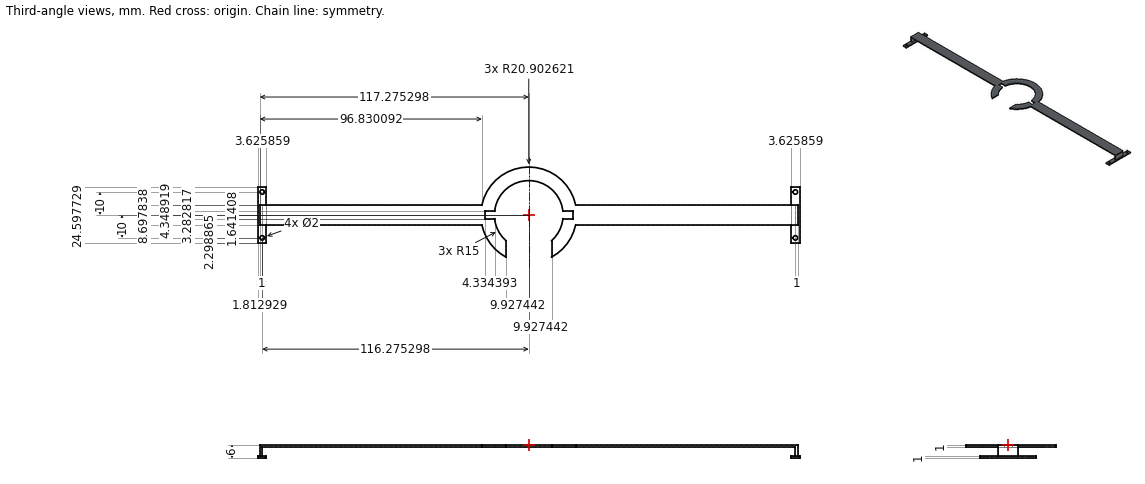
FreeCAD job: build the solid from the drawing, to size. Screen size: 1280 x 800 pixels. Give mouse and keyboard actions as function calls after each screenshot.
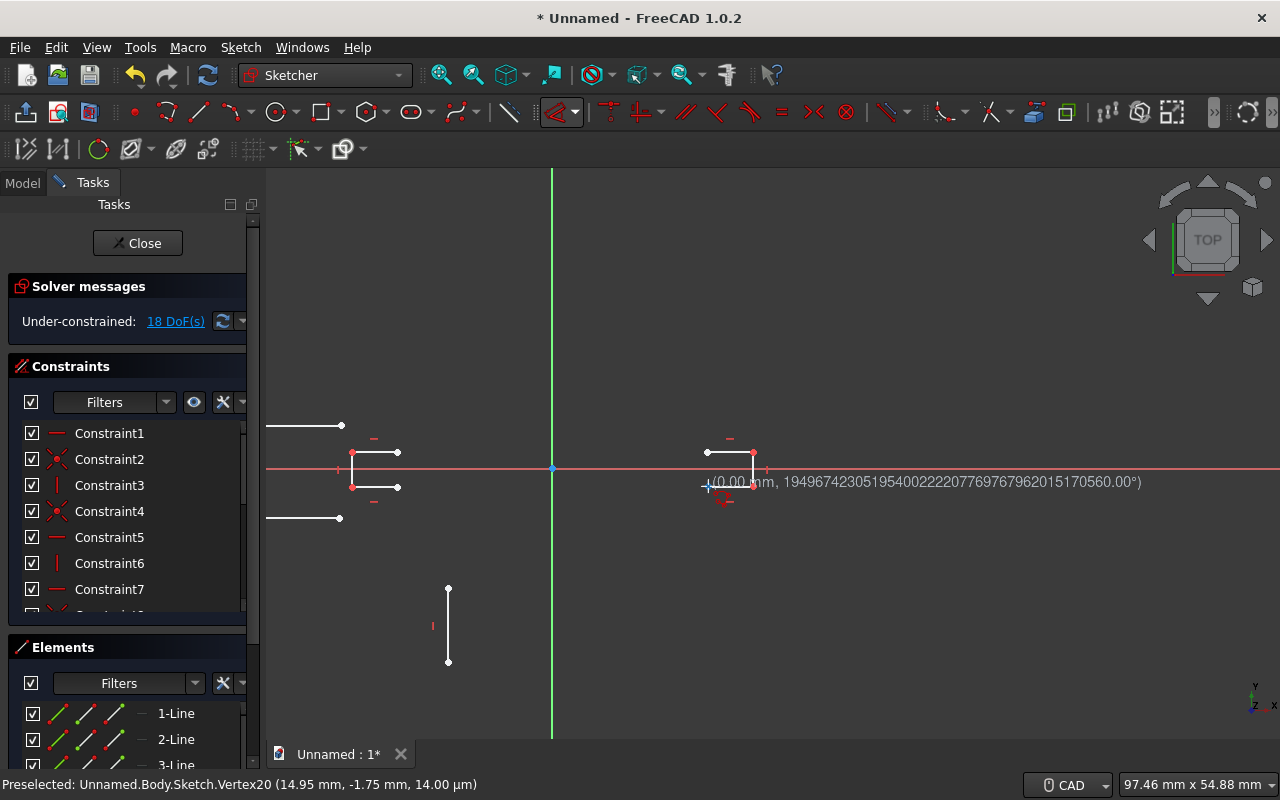
click(200, 112)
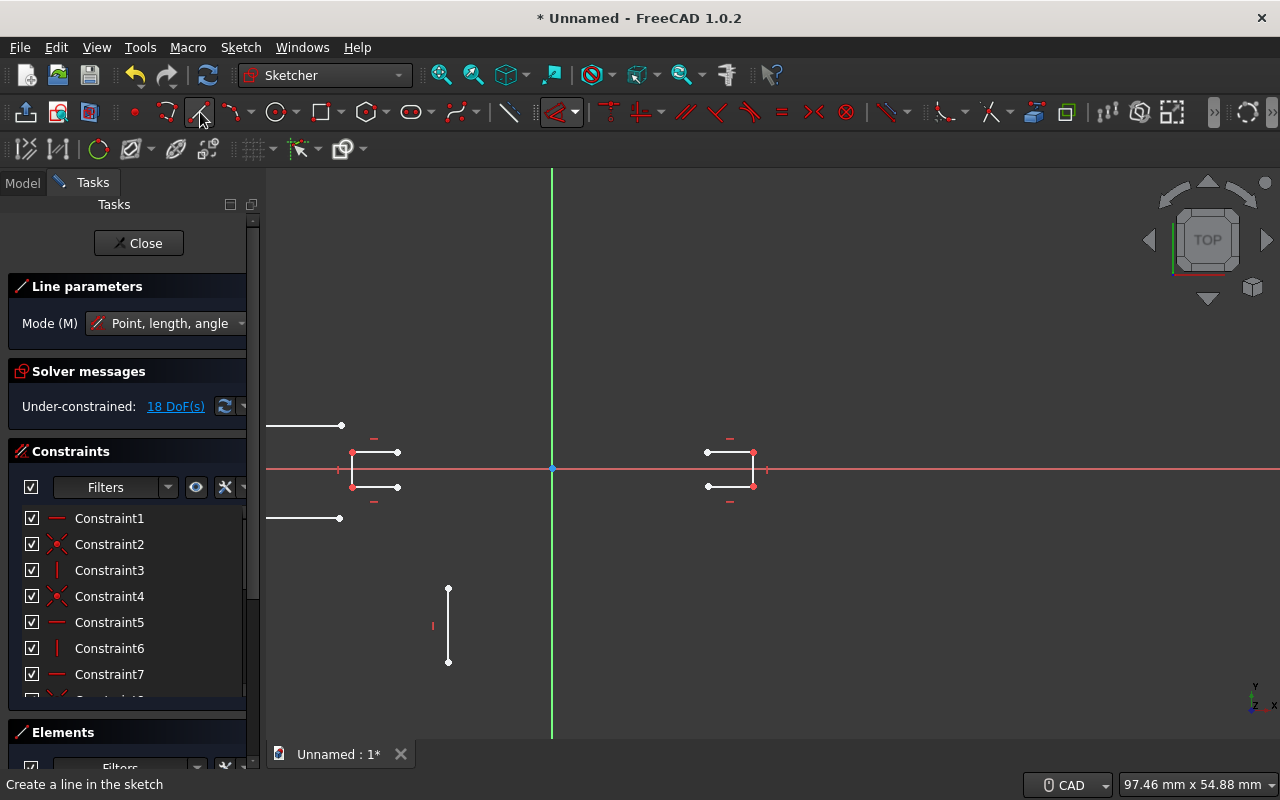
scroll(754, 453, down, 7)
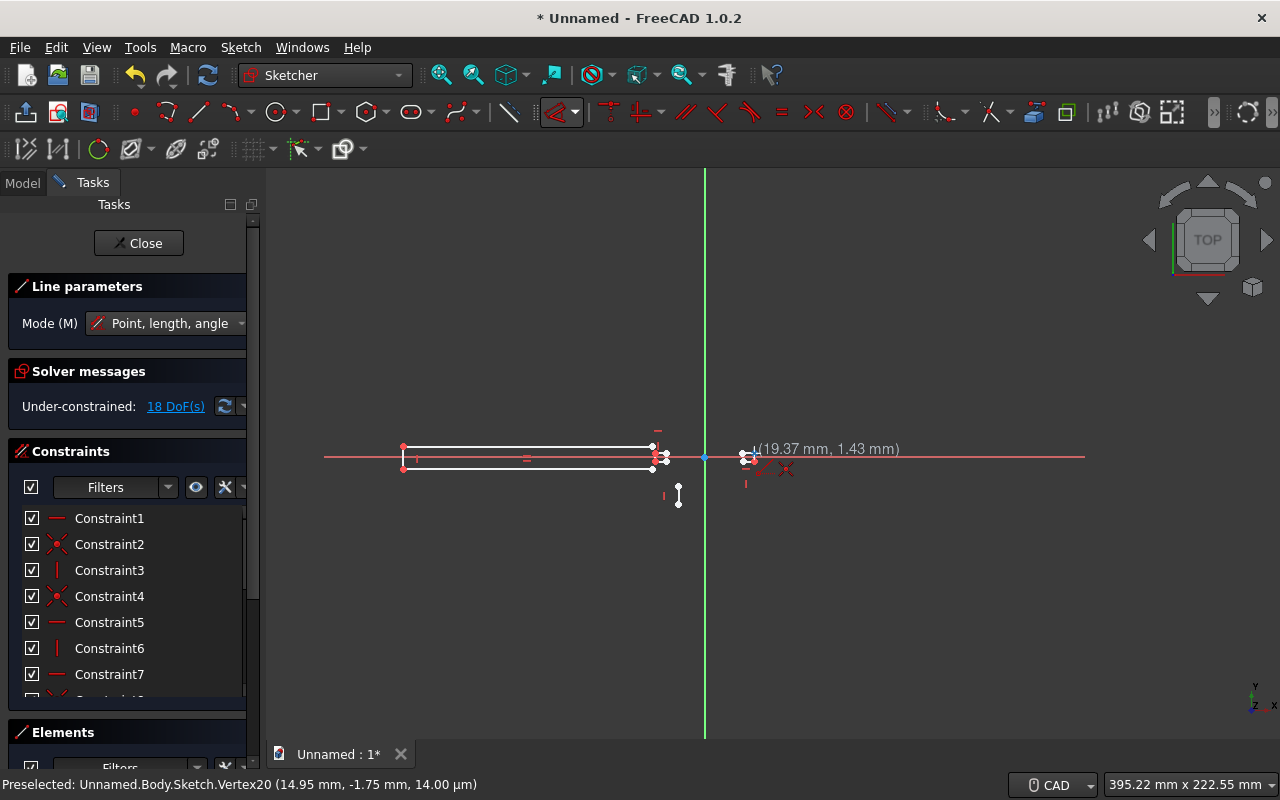
click(730, 486)
click(730, 504)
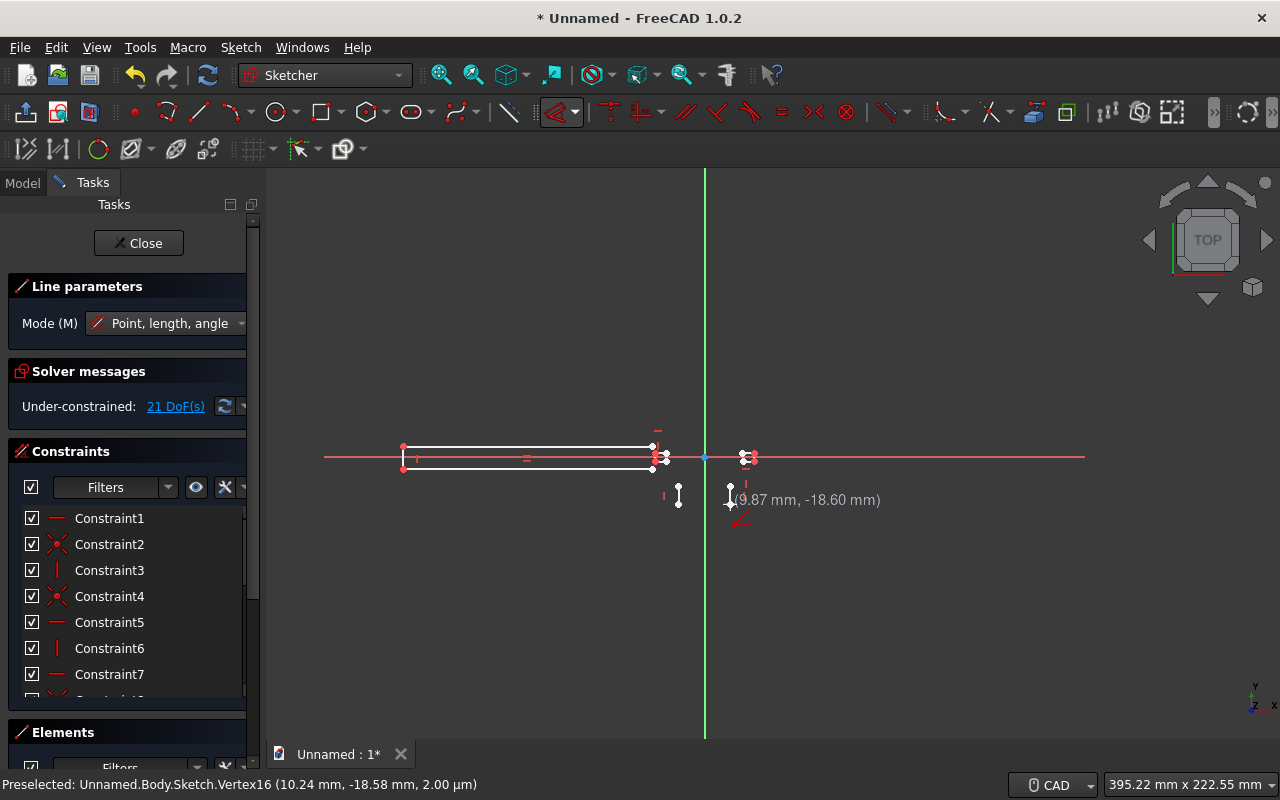
key(g)
key(m)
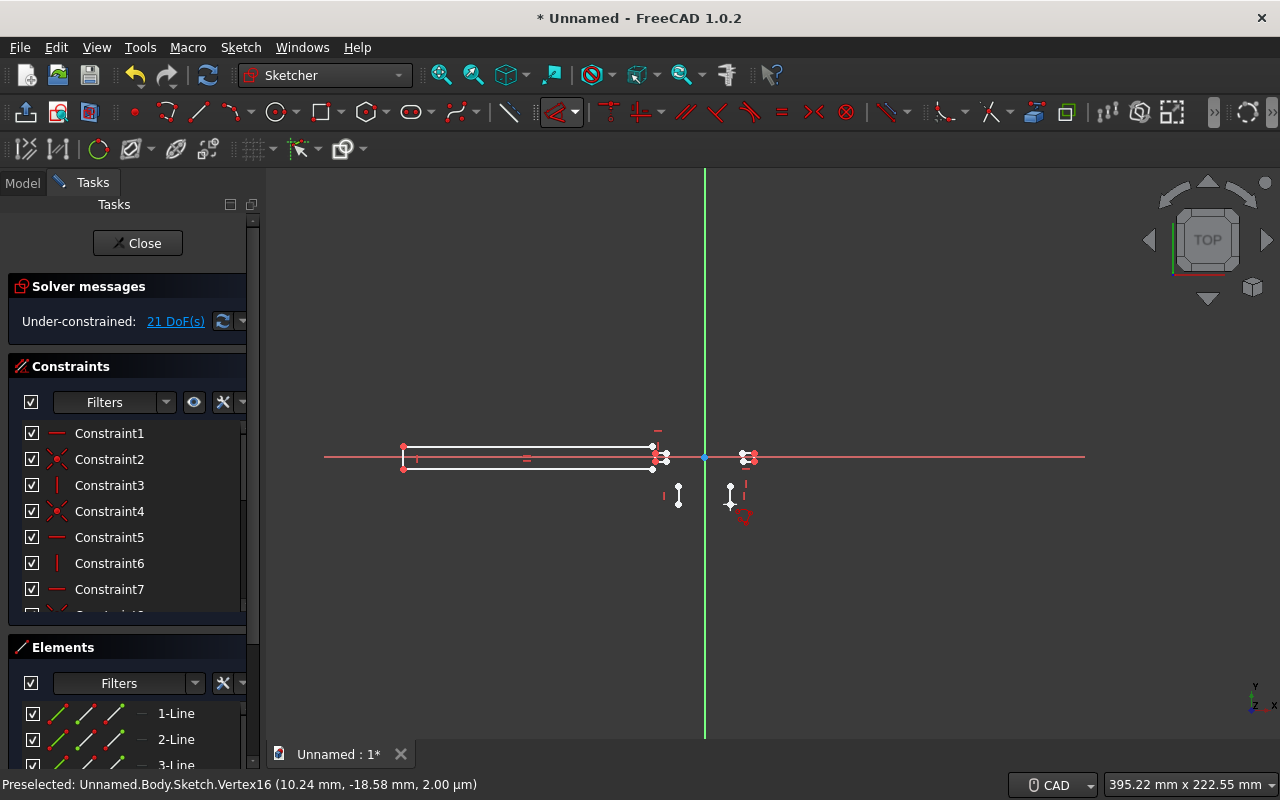
scroll(757, 468, up, 4)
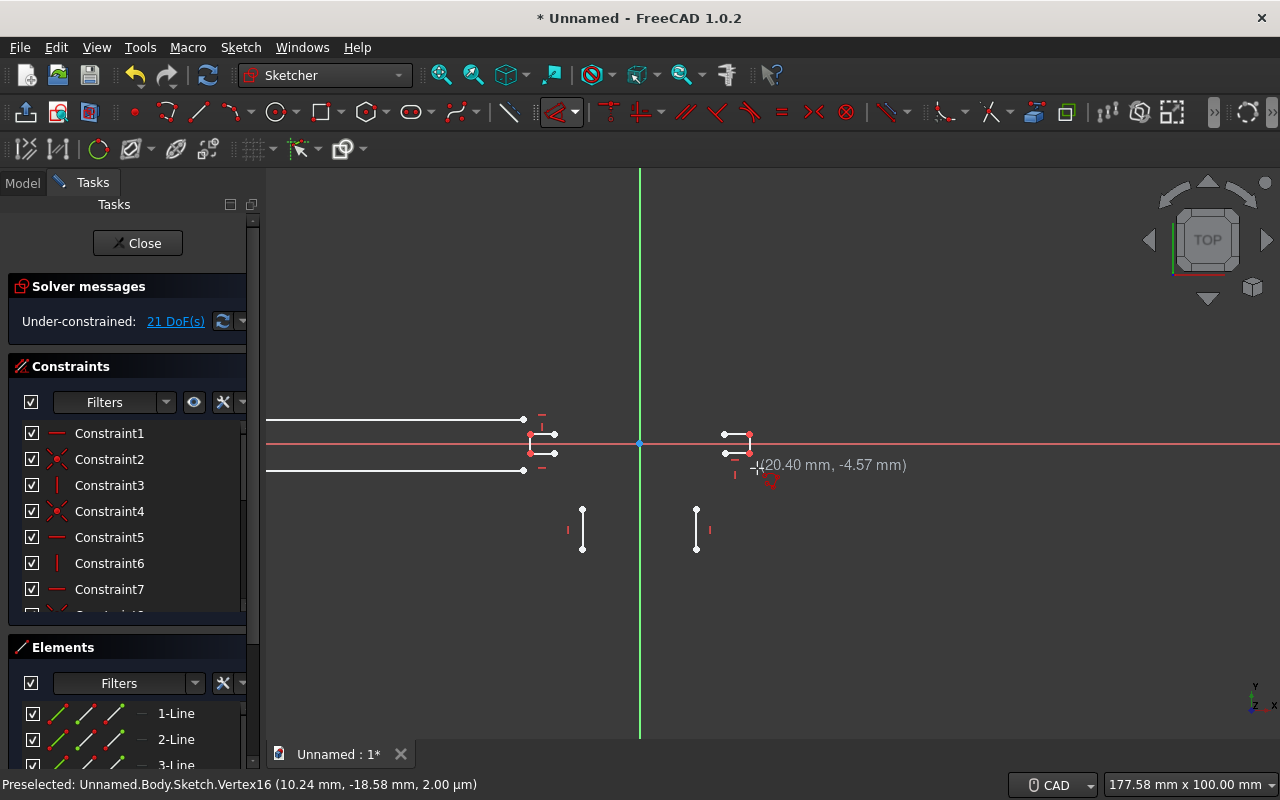
click(757, 468)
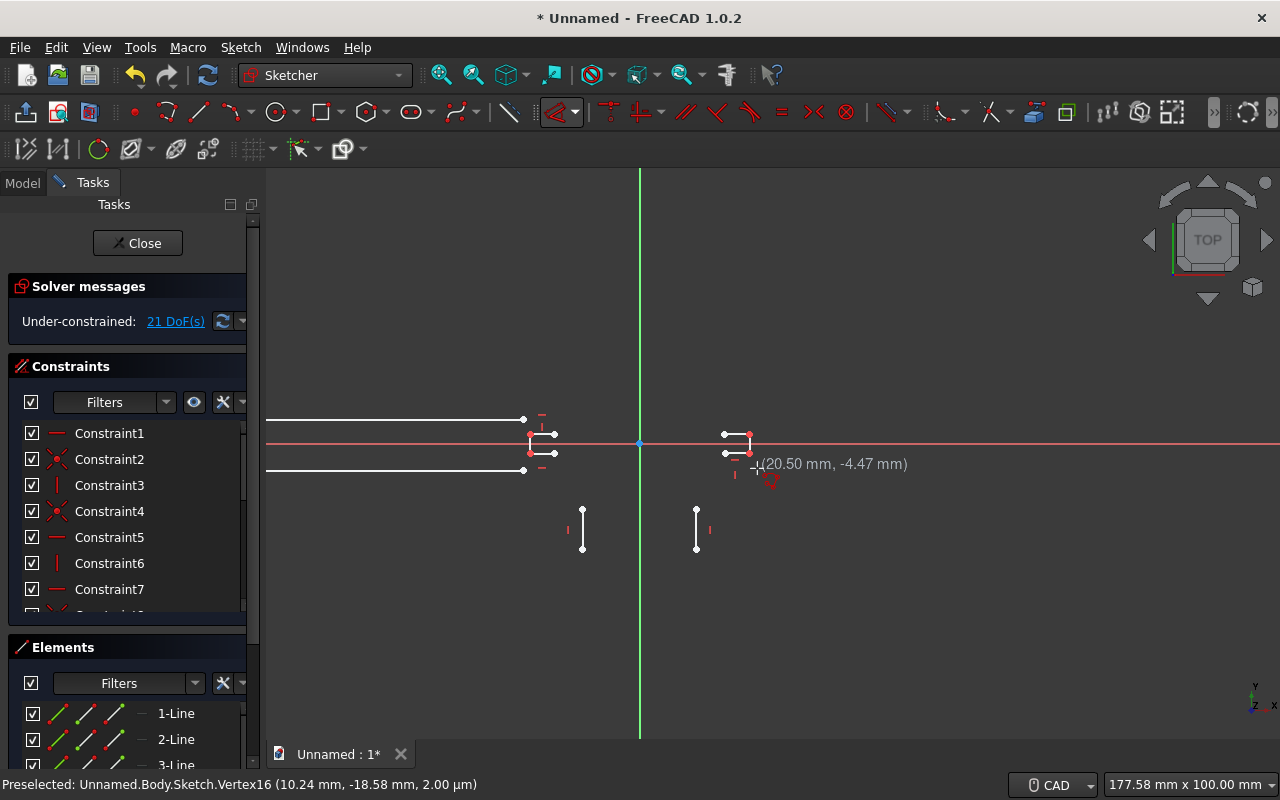
scroll(757, 467, down, 4)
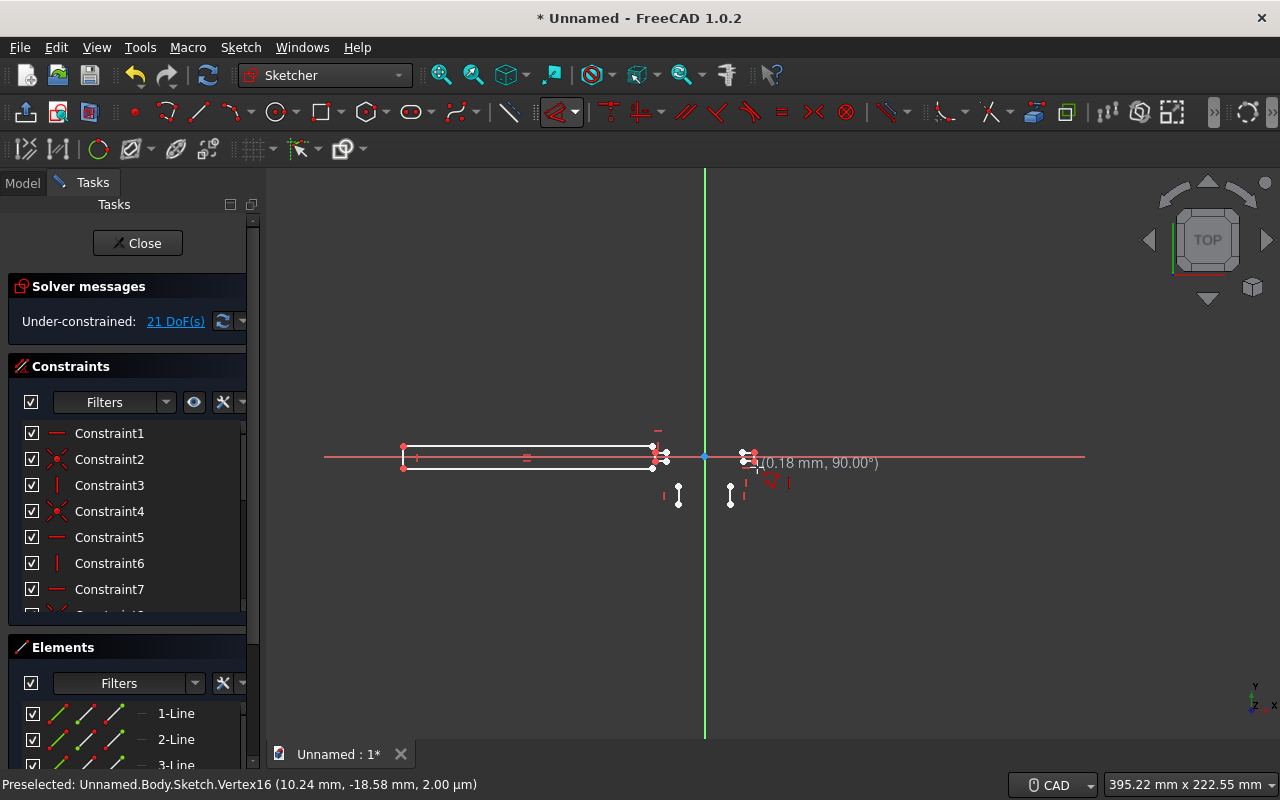
scroll(1006, 468, up, 2)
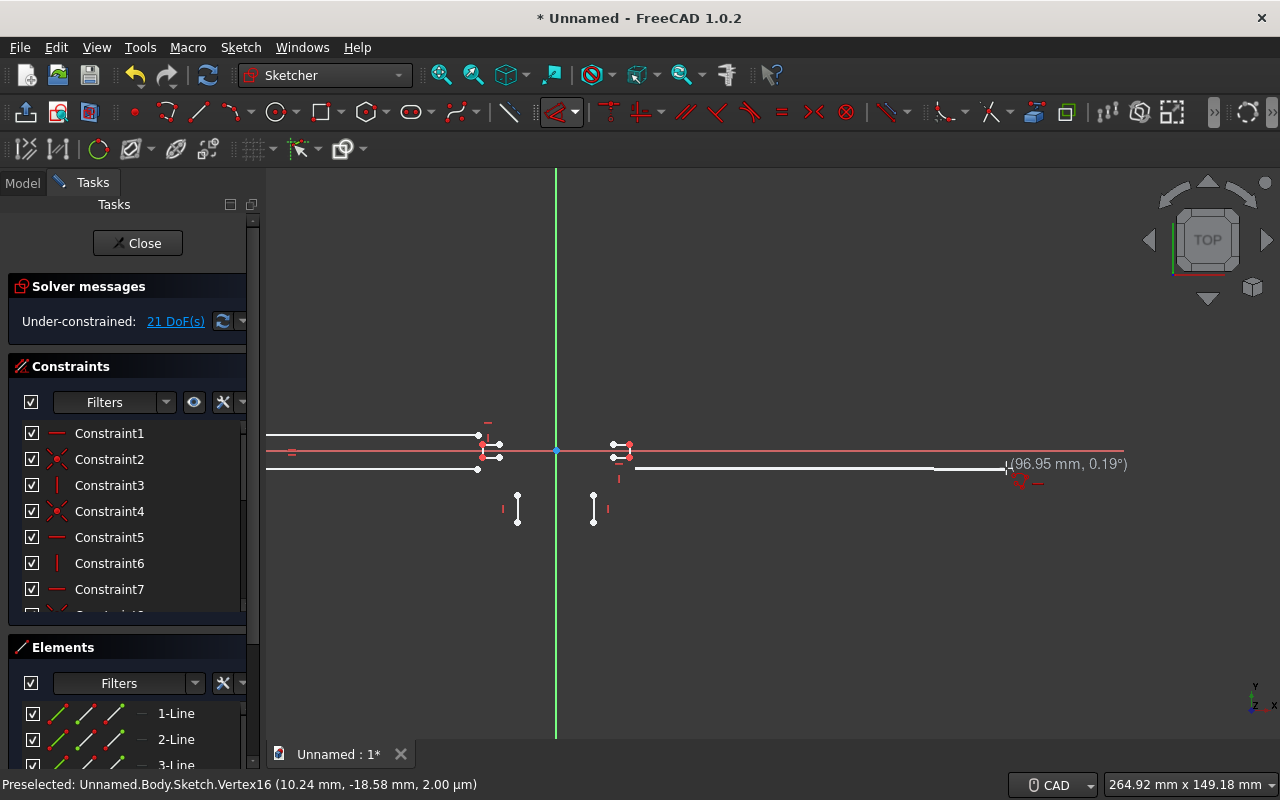
click(1005, 467)
click(1005, 434)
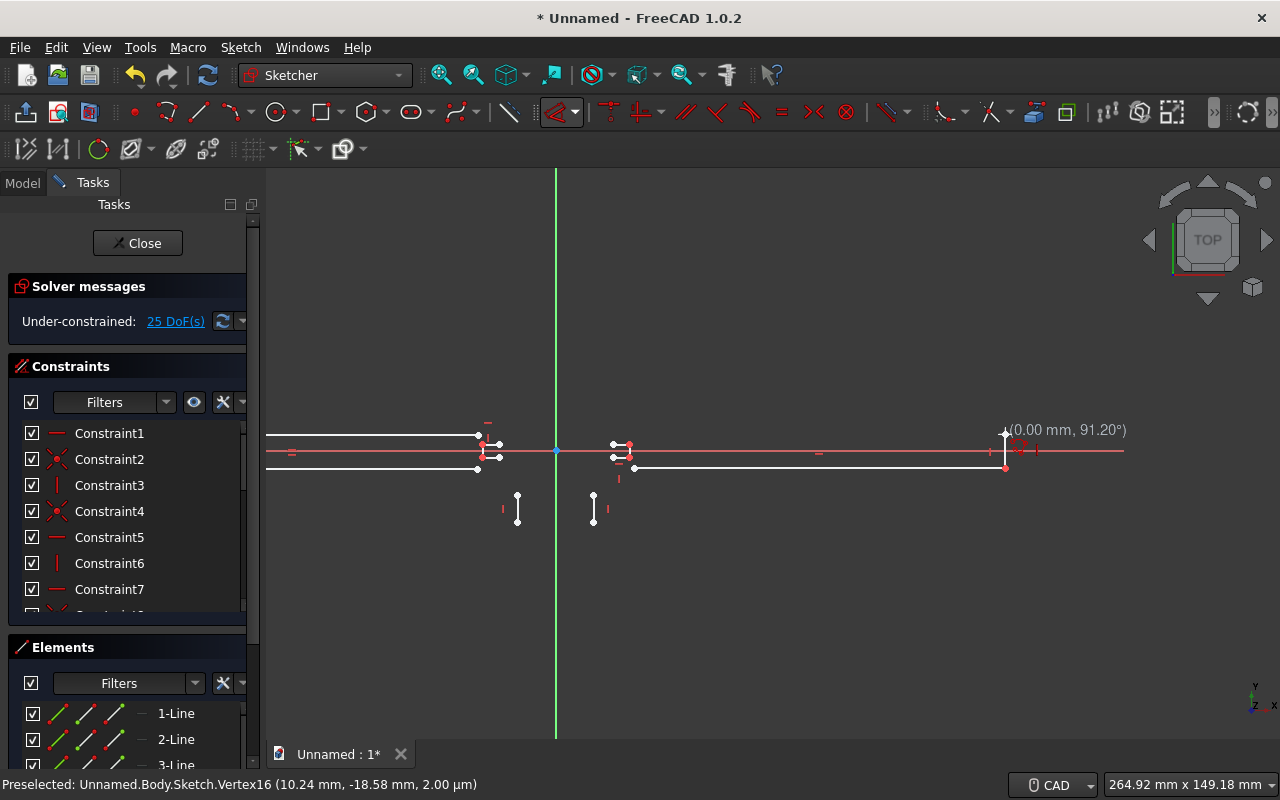
scroll(634, 434, up, 2)